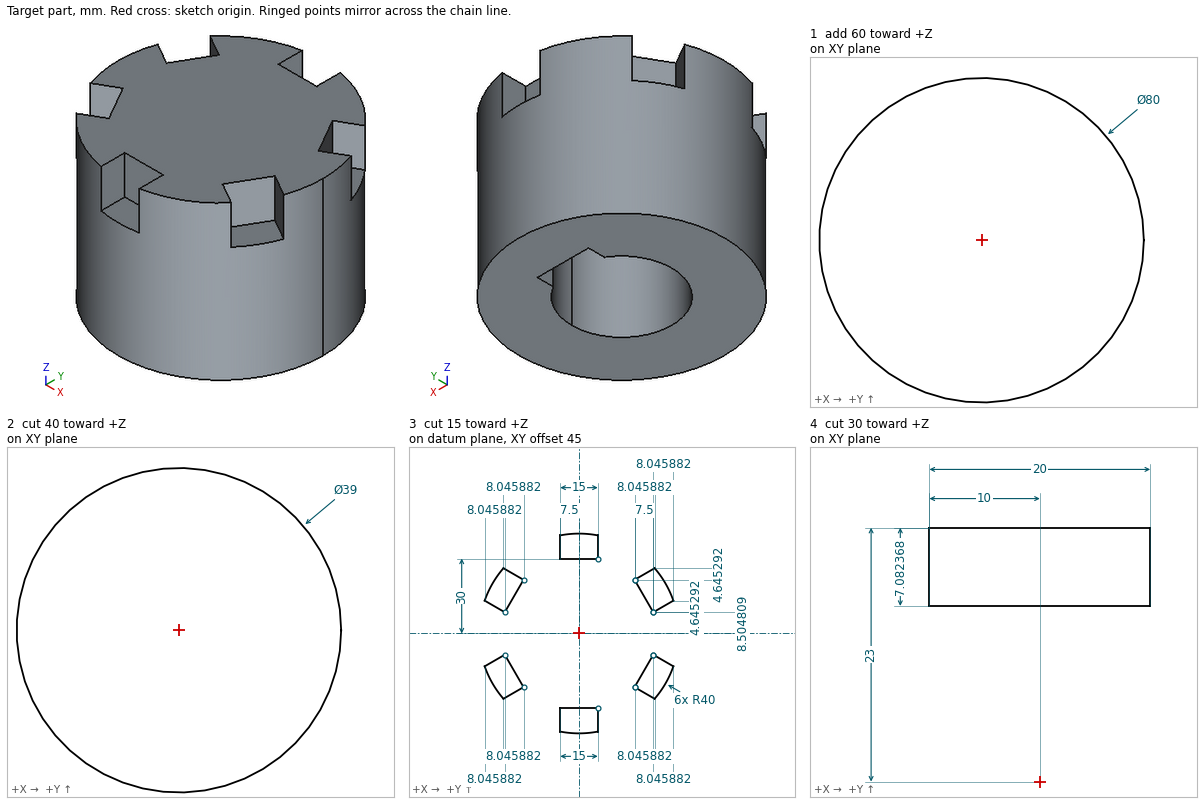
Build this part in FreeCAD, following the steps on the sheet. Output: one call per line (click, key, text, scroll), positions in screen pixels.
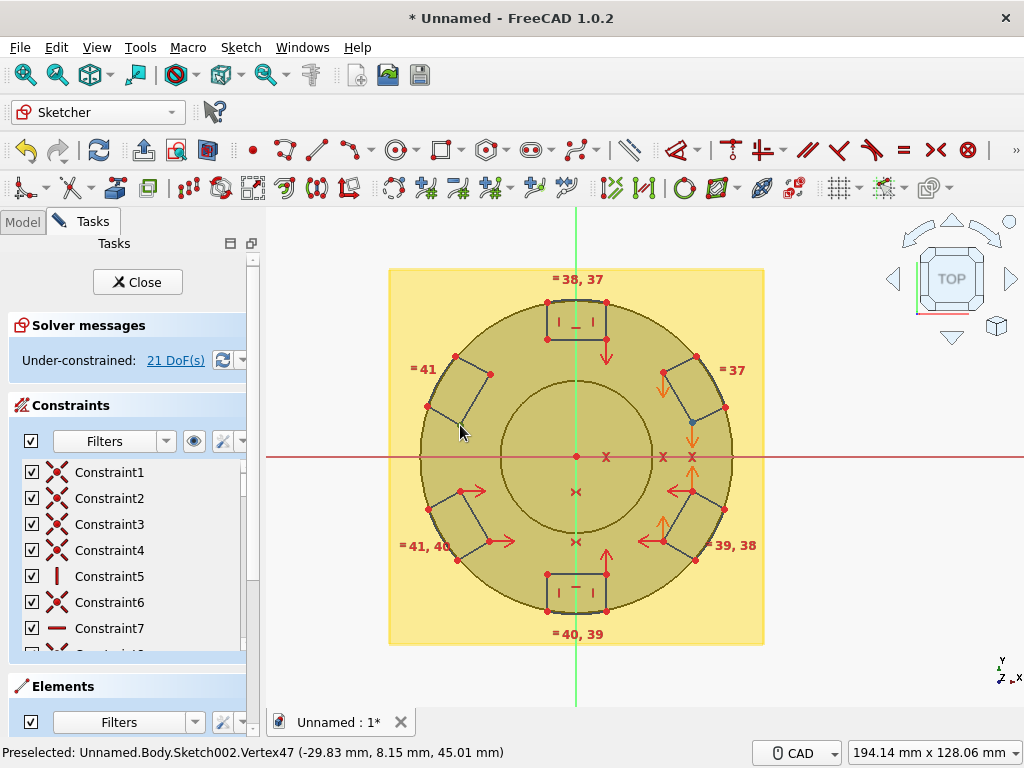
click(576, 647)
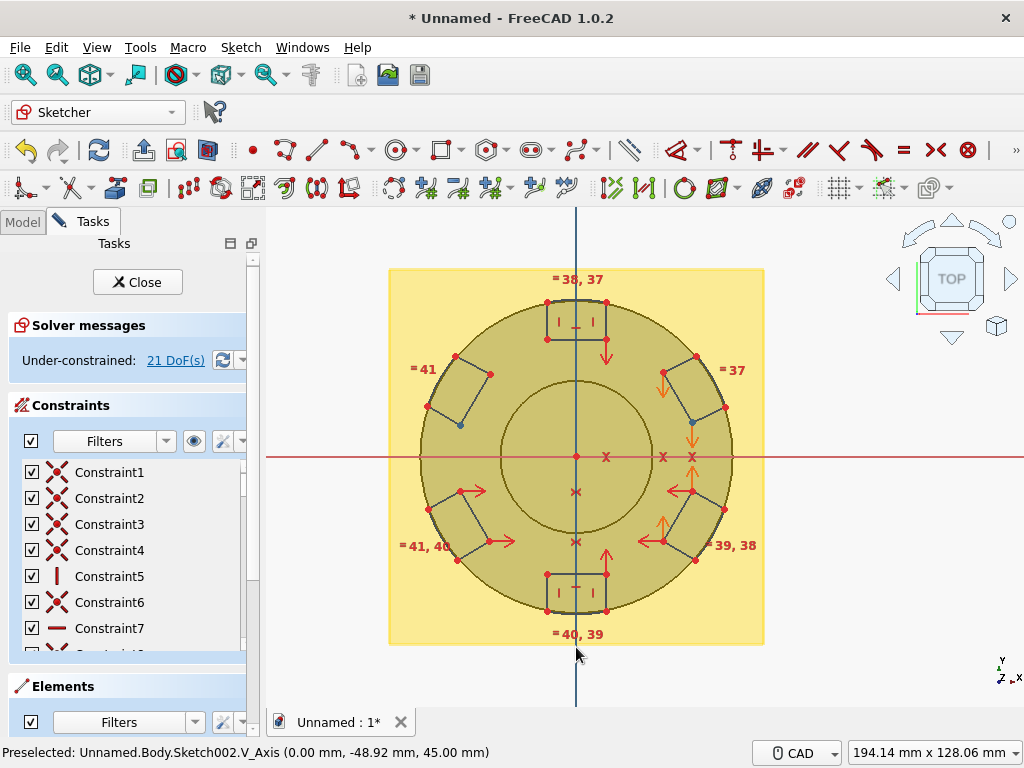
click(936, 150)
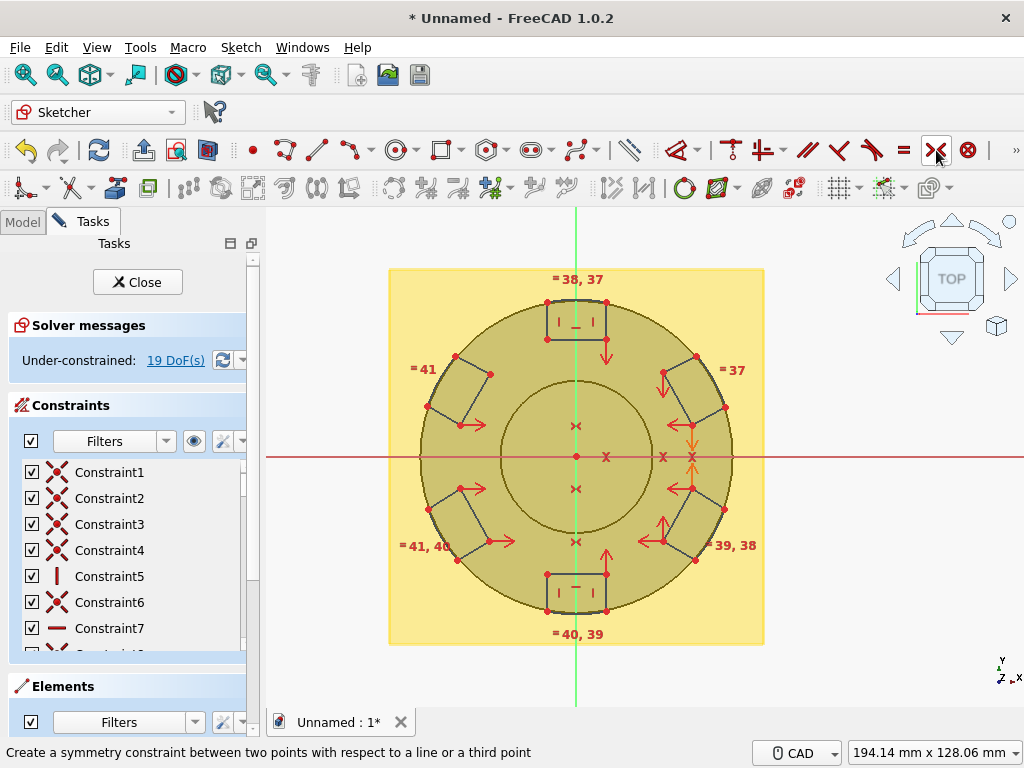
click(663, 373)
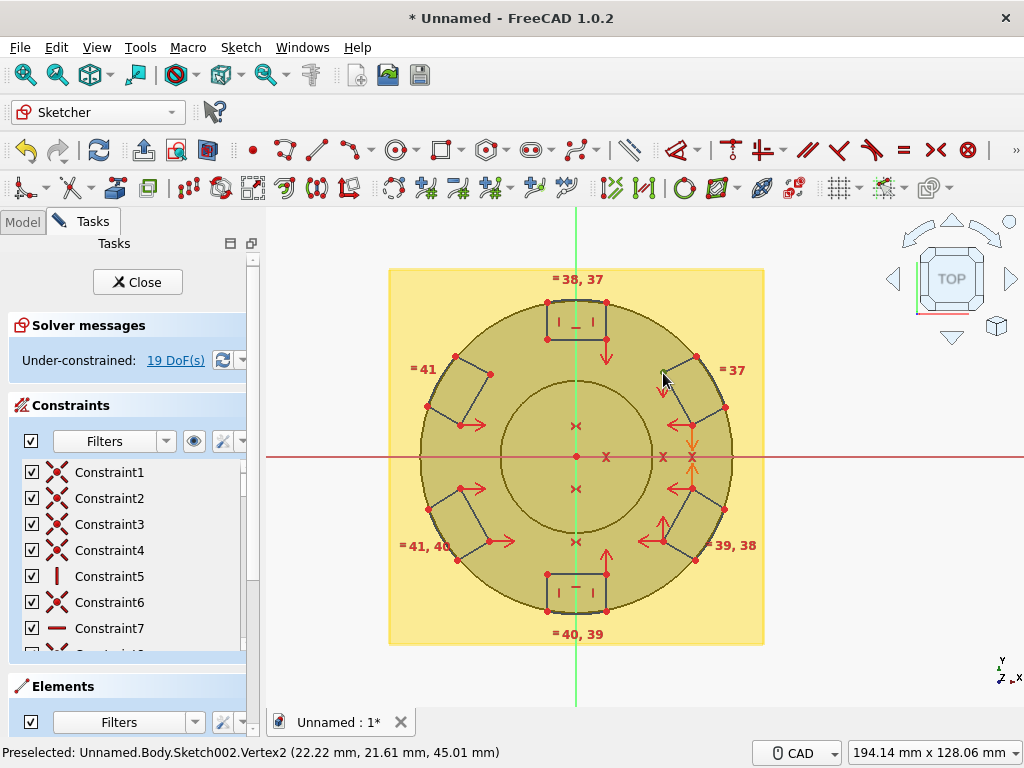
click(490, 374)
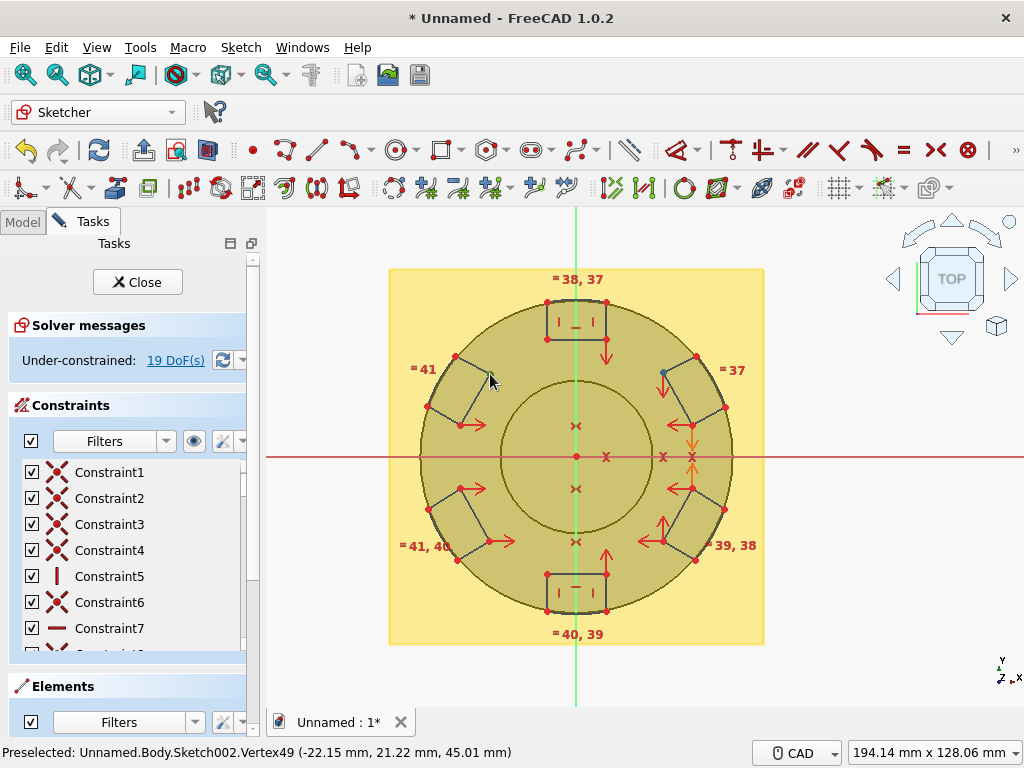
click(576, 647)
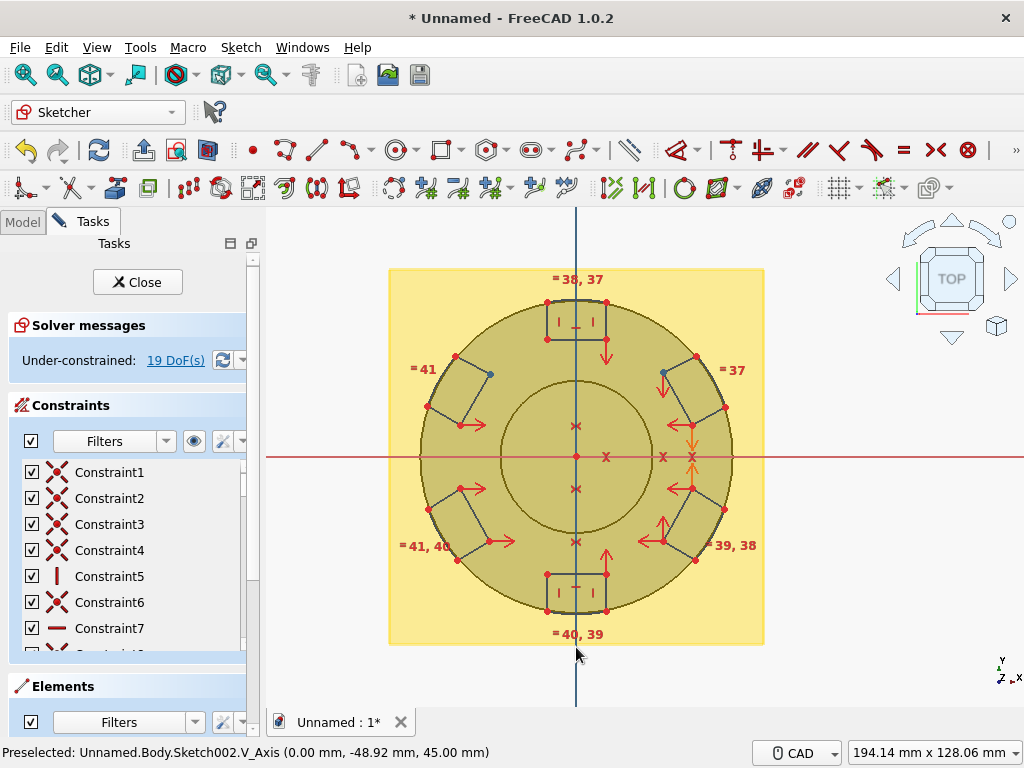
click(936, 150)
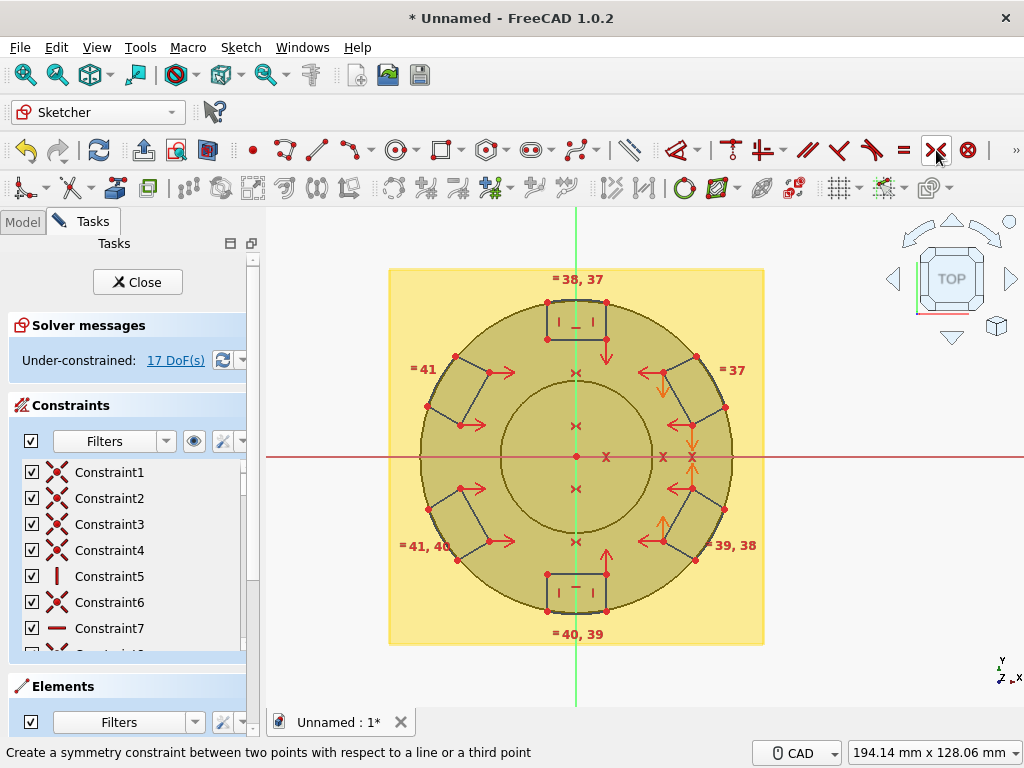
click(676, 150)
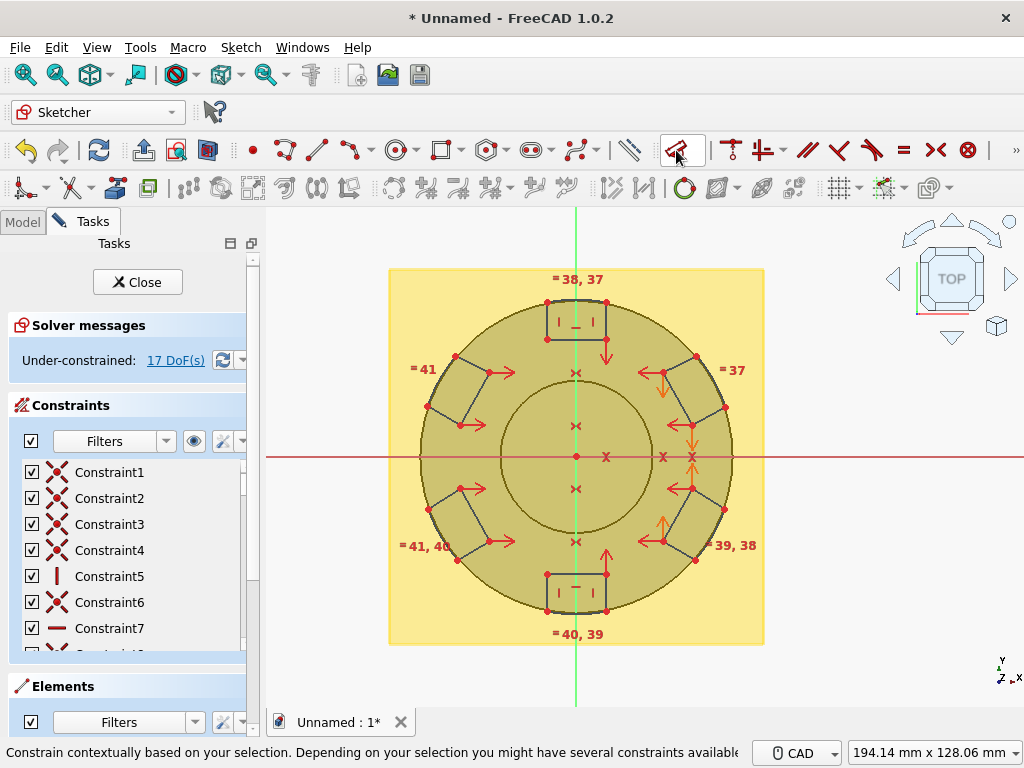
click(719, 391)
click(748, 378)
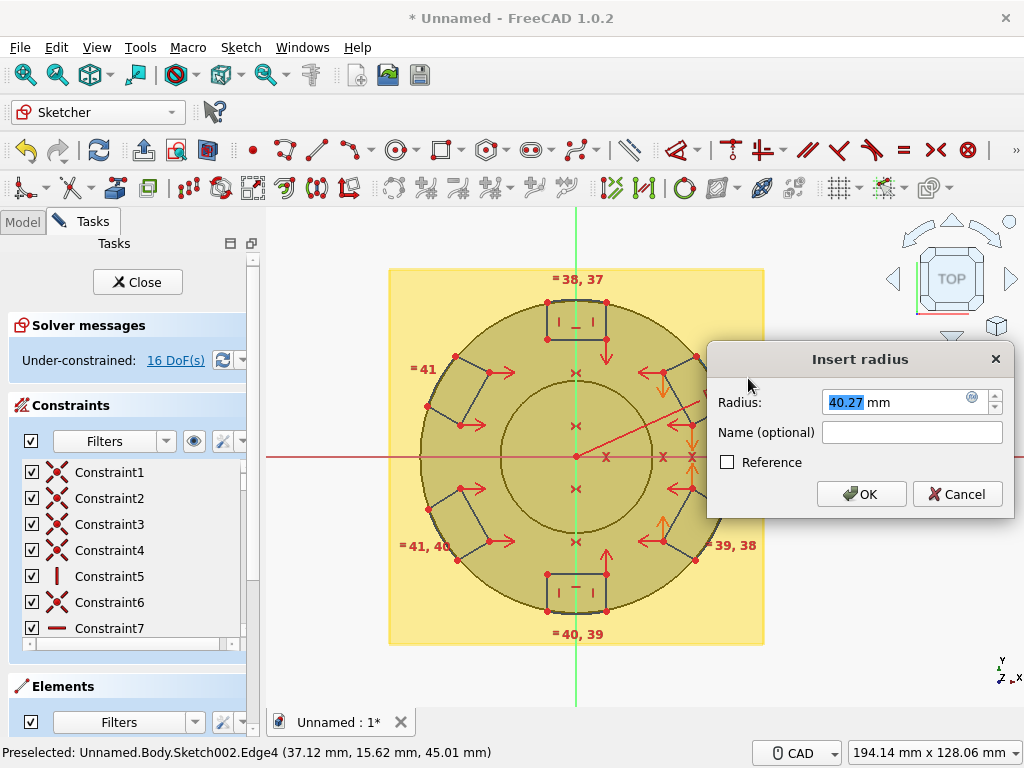
text(40)
key(Return)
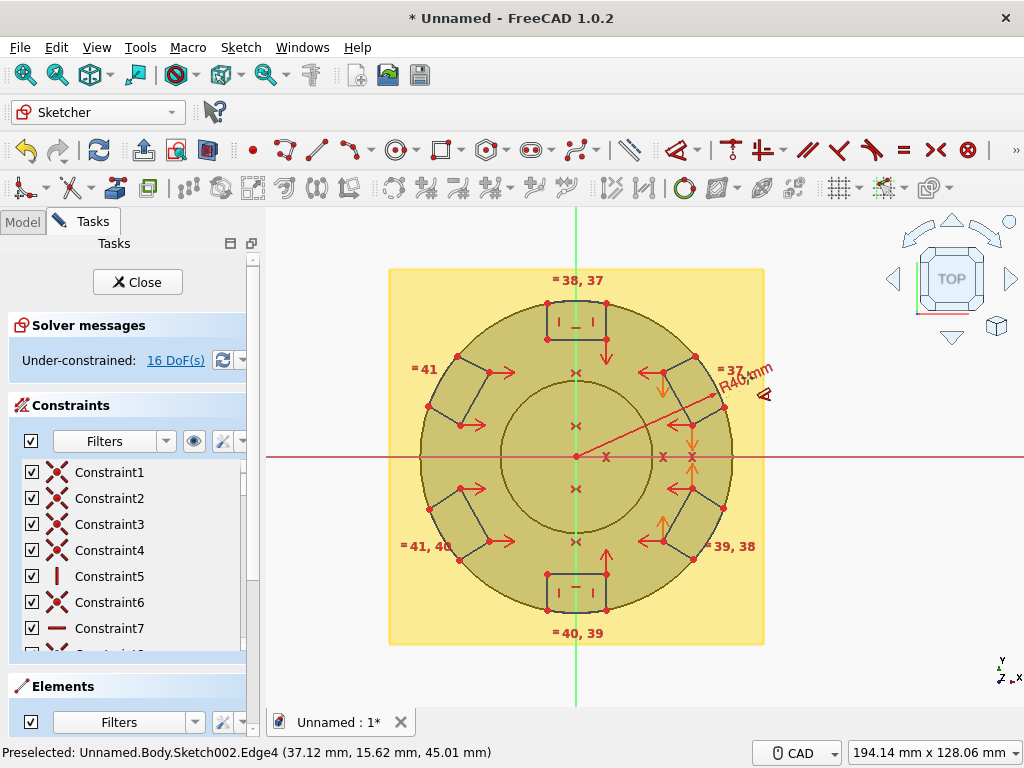
click(565, 340)
click(563, 374)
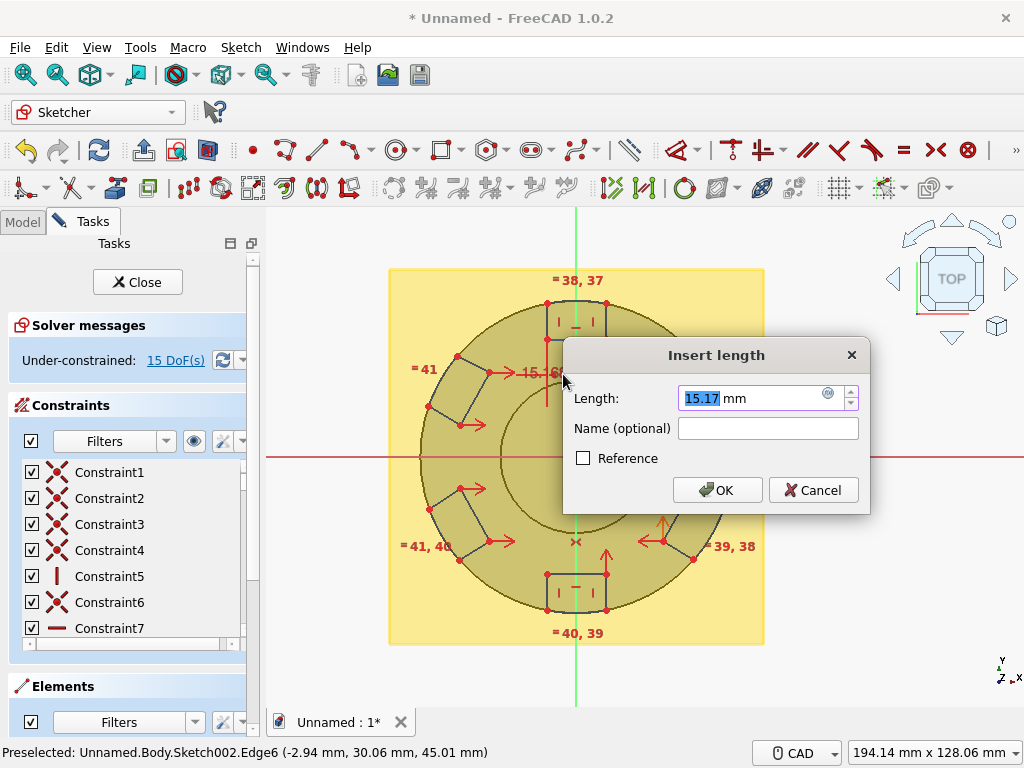
text(15)
key(Return)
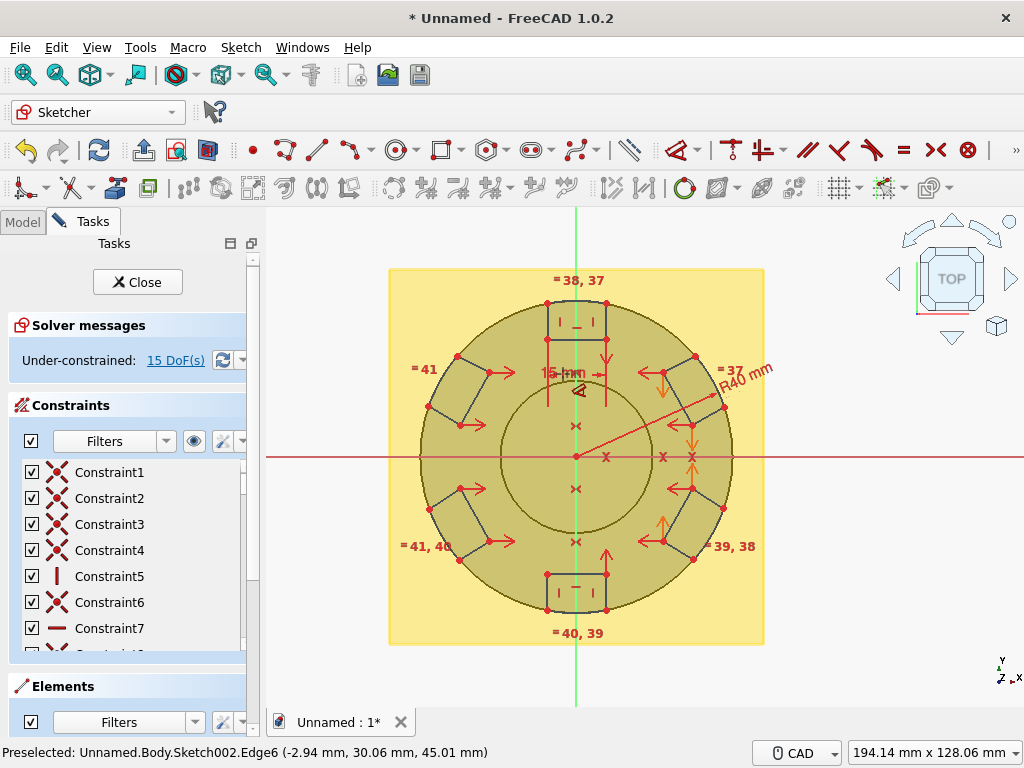
click(589, 574)
click(563, 540)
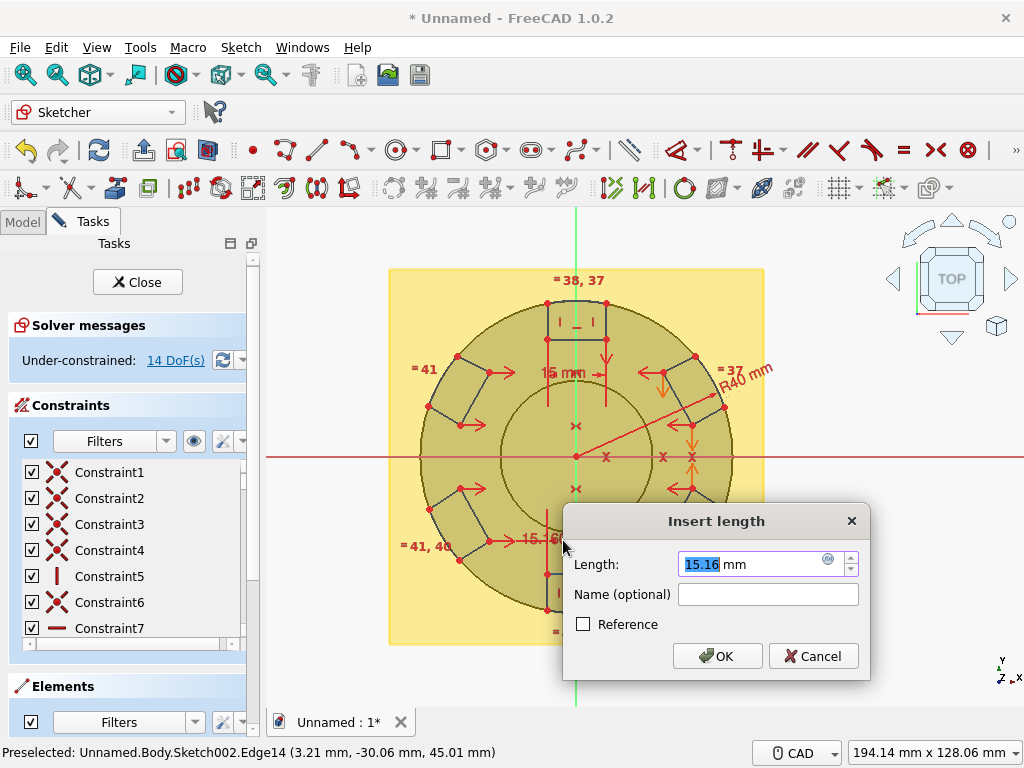
text(15)
key(Return)